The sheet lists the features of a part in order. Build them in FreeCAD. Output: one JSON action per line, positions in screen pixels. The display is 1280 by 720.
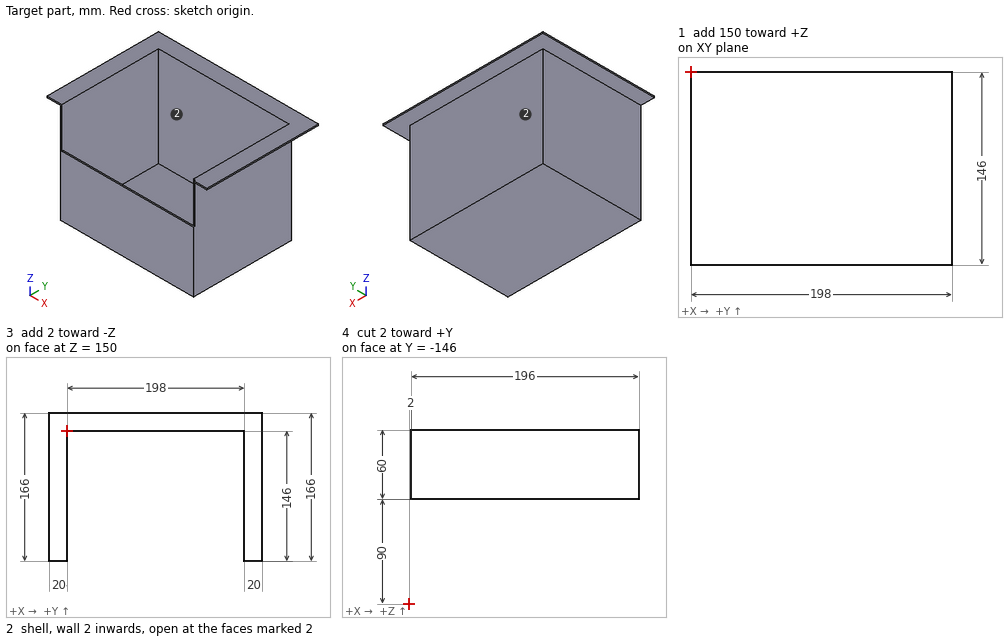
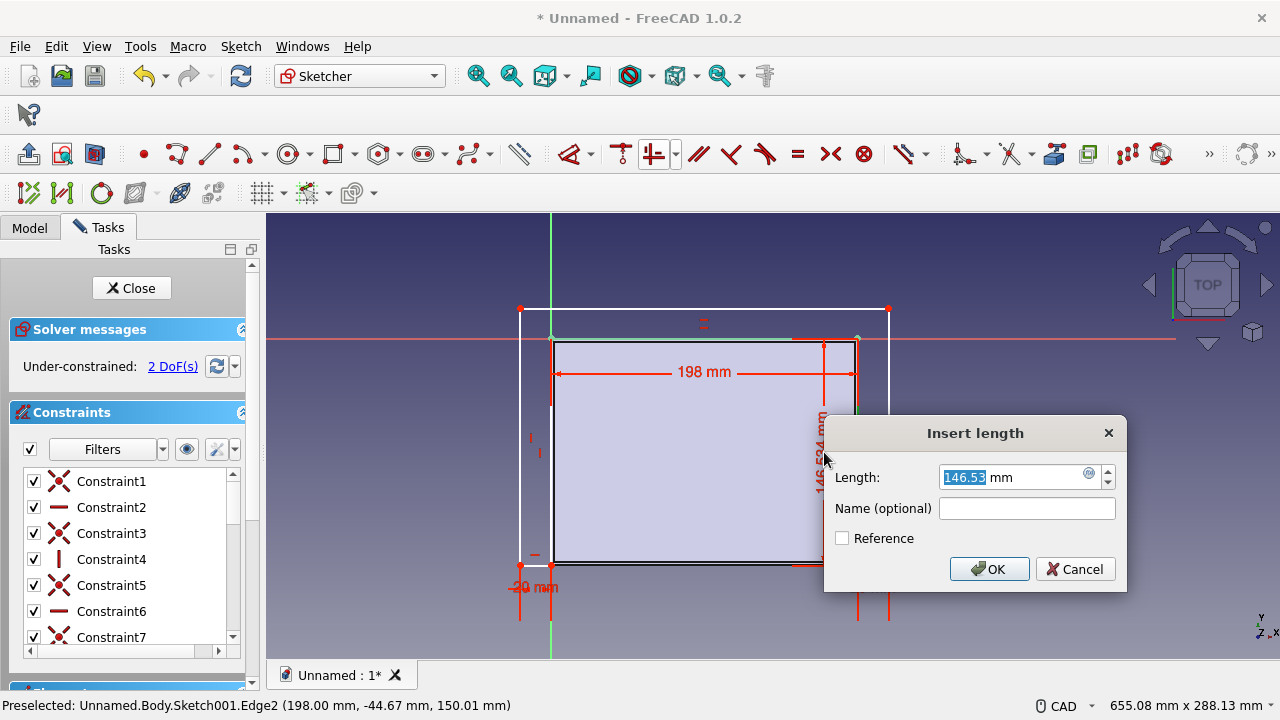
{"action": "type", "text": "146"}
{"action": "key", "text": "Return"}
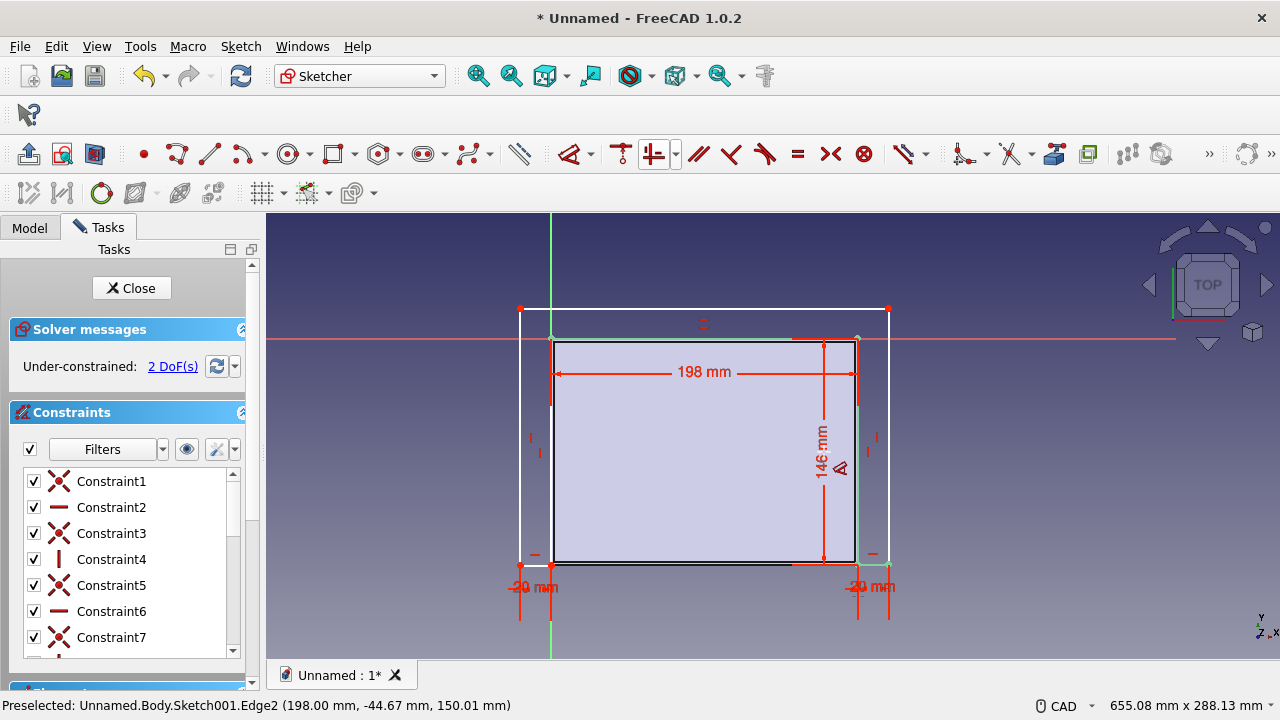
{"action": "left_click", "coordinate": [889, 488]}
{"action": "left_click", "coordinate": [923, 437]}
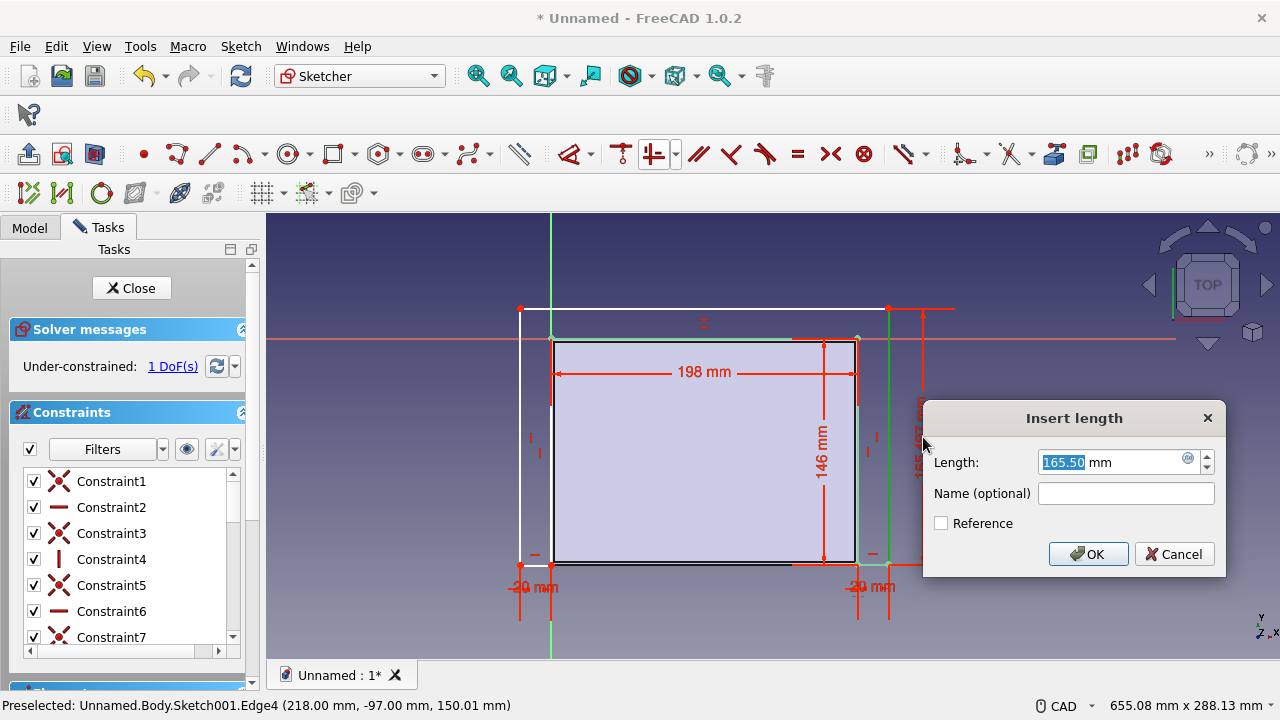
{"action": "type", "text": "166"}
{"action": "key", "text": "Return"}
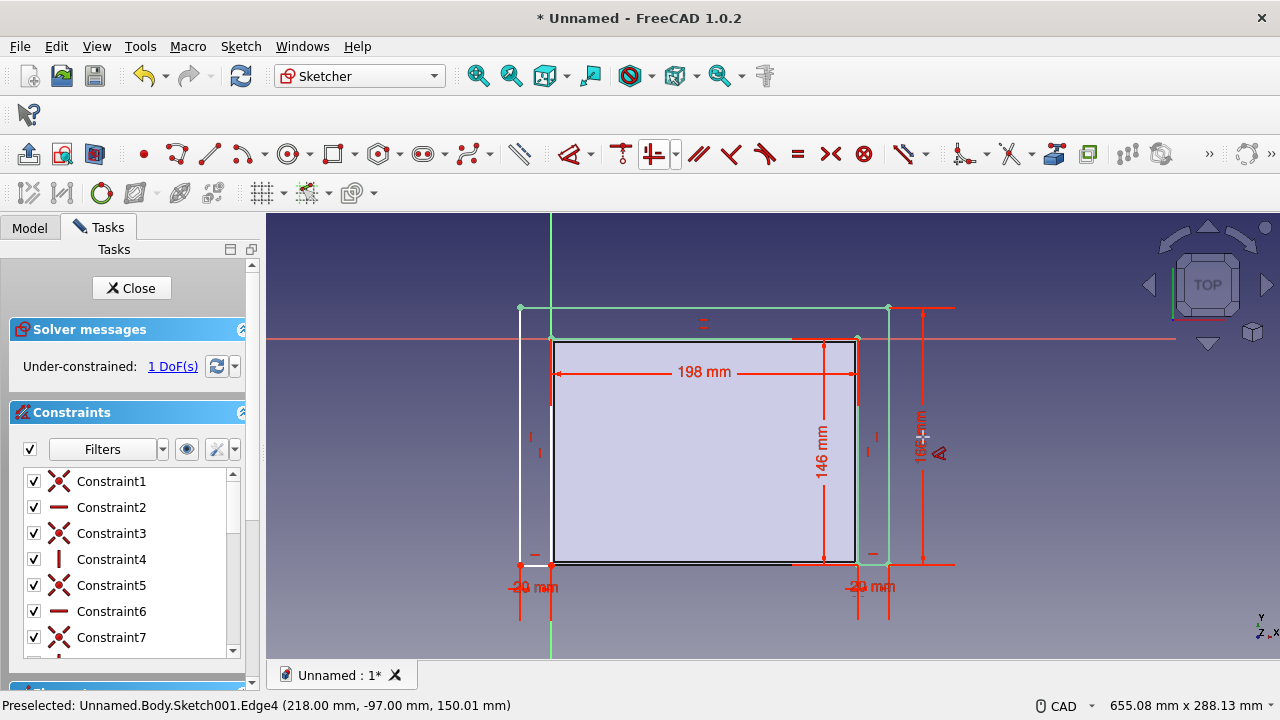
{"action": "left_click", "coordinate": [520, 385]}
{"action": "left_click", "coordinate": [486, 437]}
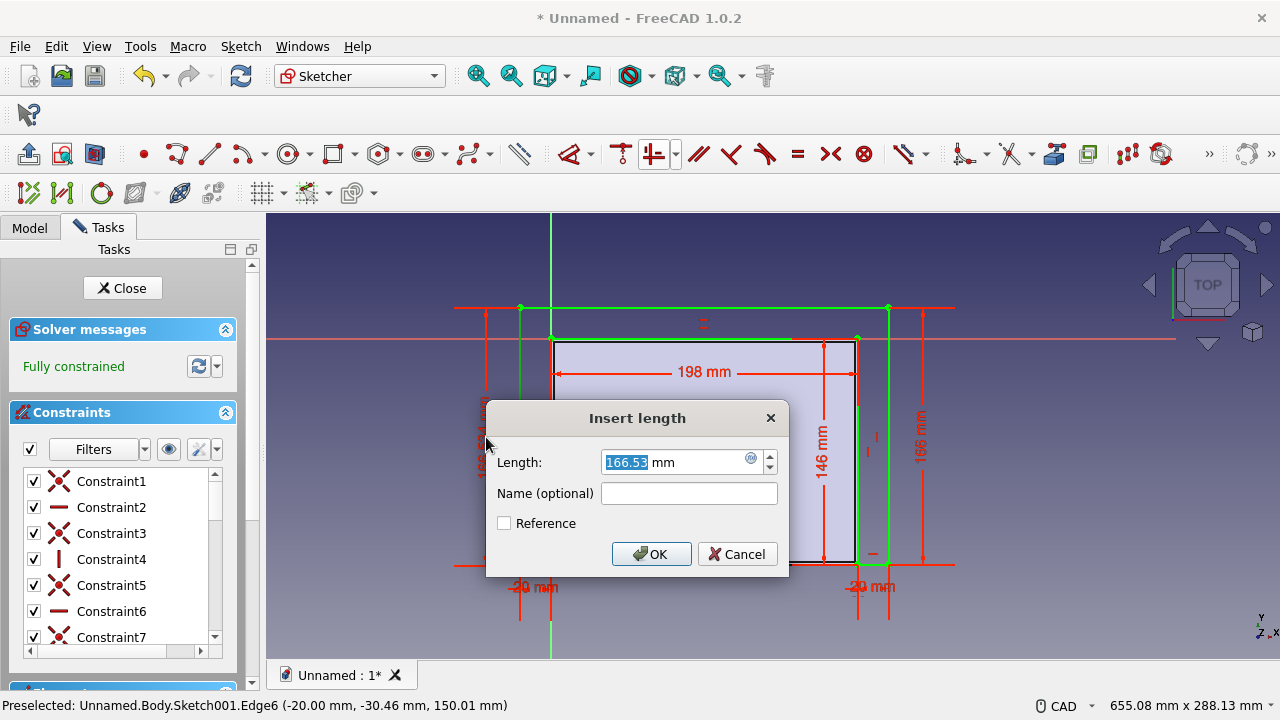
{"action": "type", "text": "166"}
{"action": "key", "text": "Return"}
{"action": "key", "text": "Escape"}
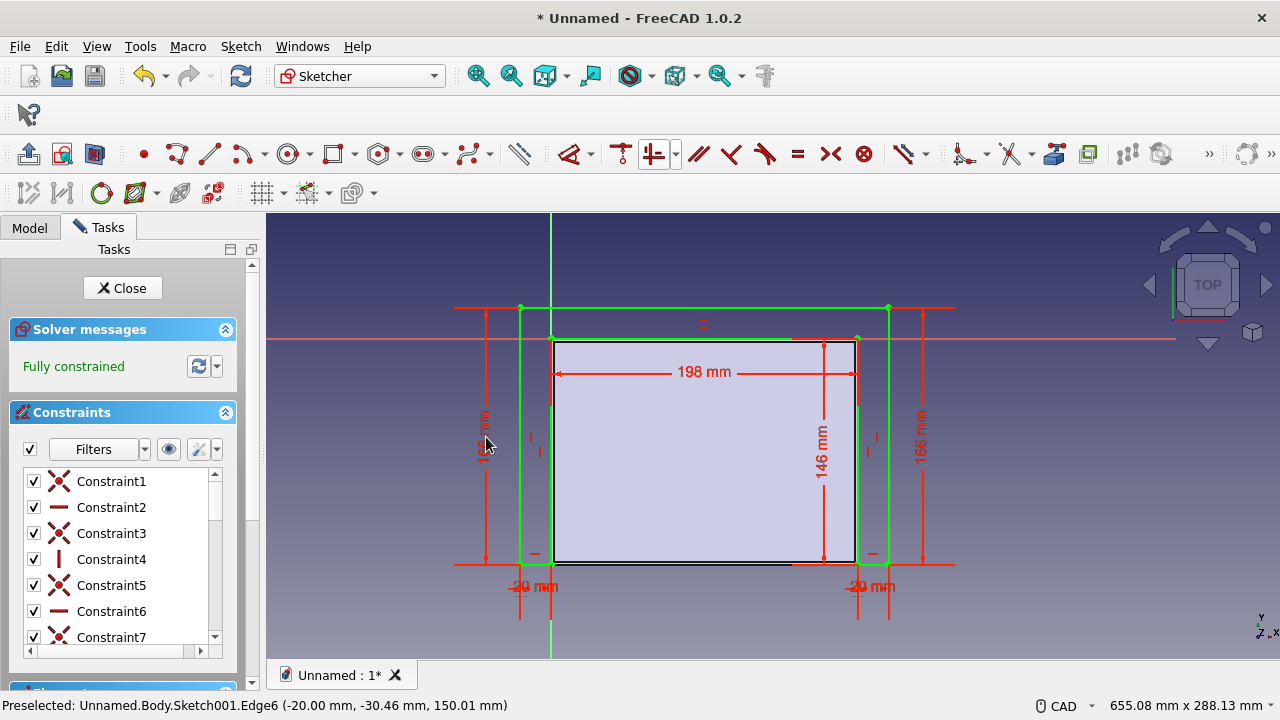
{"action": "left_click", "coordinate": [123, 288]}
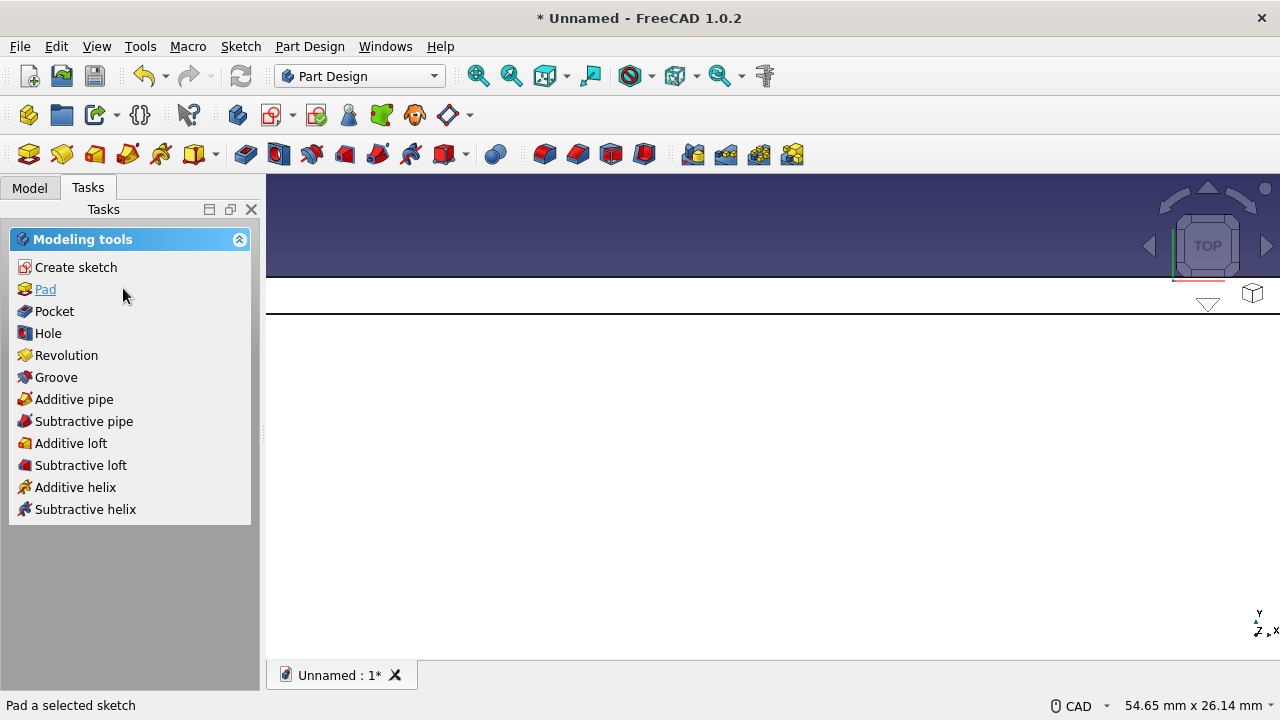
{"action": "left_click", "coordinate": [29, 154]}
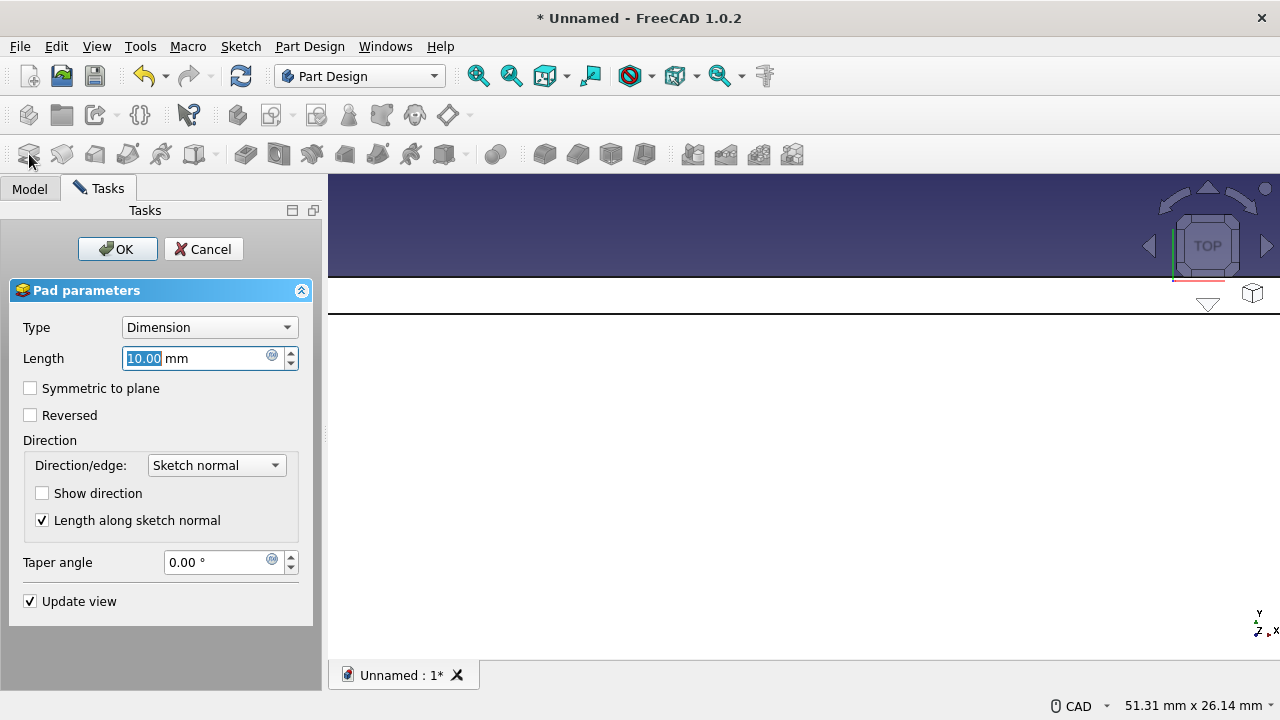
{"action": "type", "text": "2"}
{"action": "key", "text": "Tab"}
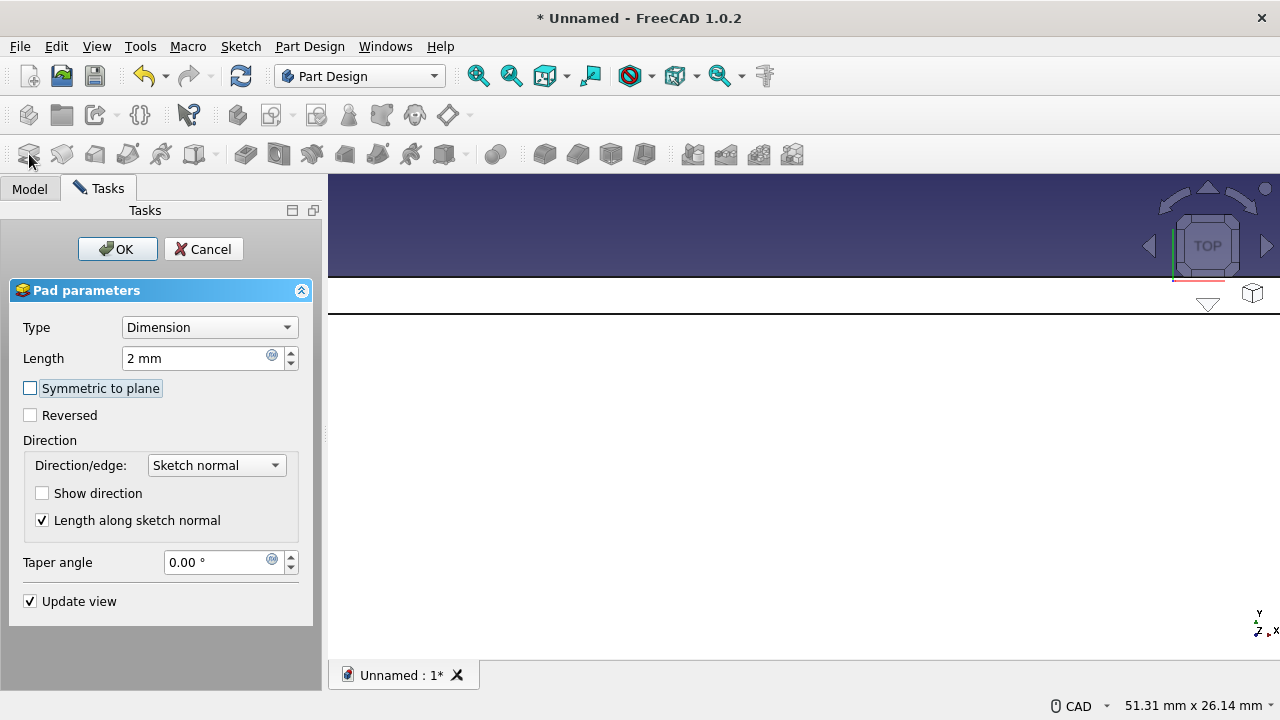
{"action": "left_click", "coordinate": [31, 415]}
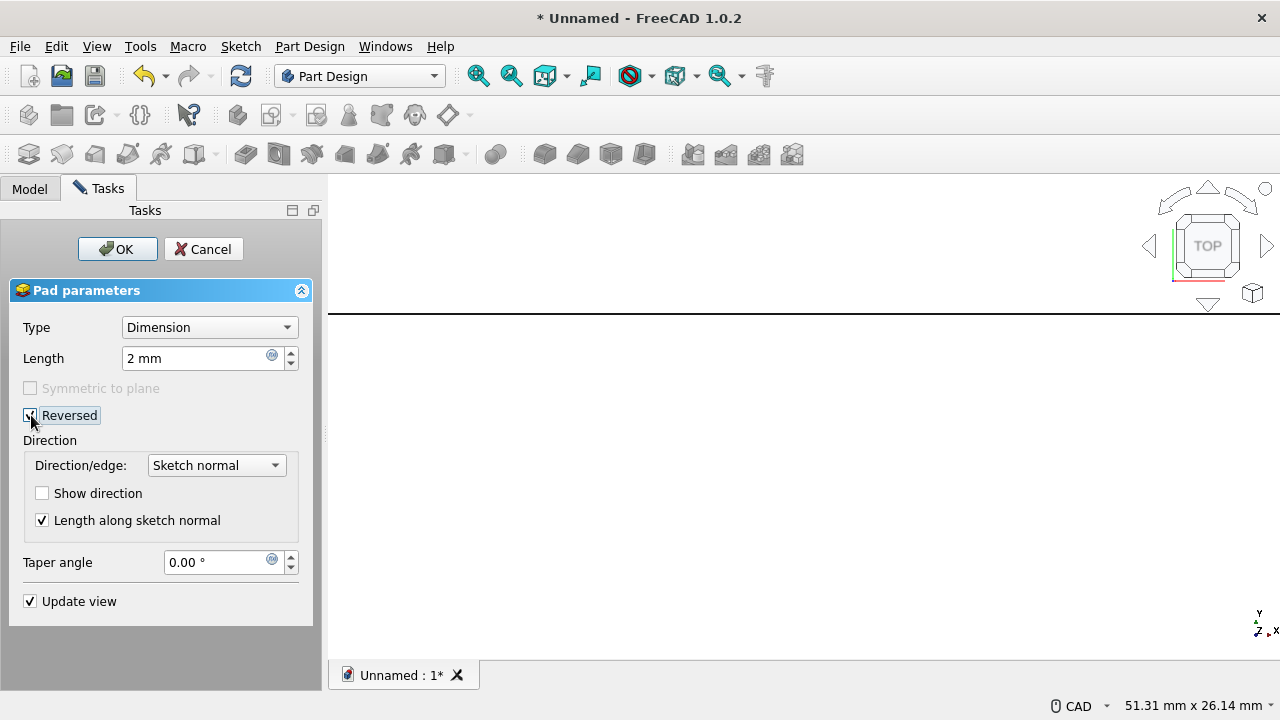
{"action": "left_click", "coordinate": [118, 249]}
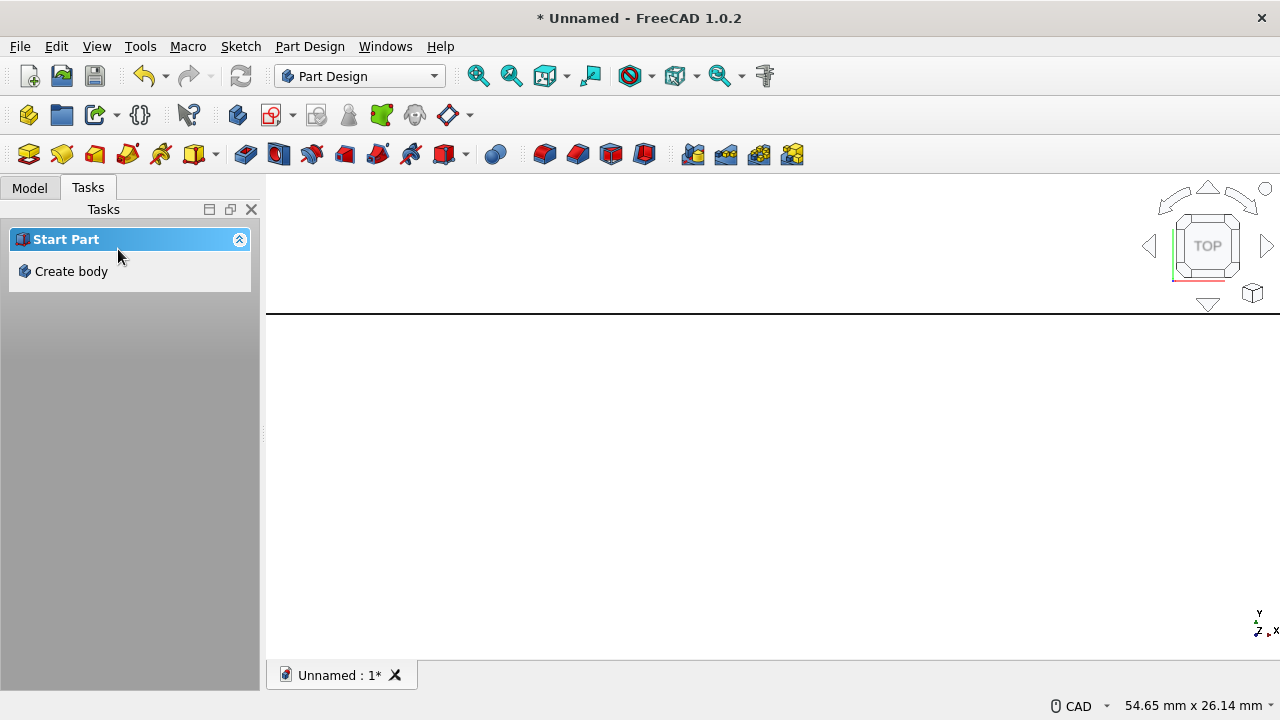
{"action": "left_click", "coordinate": [479, 76]}